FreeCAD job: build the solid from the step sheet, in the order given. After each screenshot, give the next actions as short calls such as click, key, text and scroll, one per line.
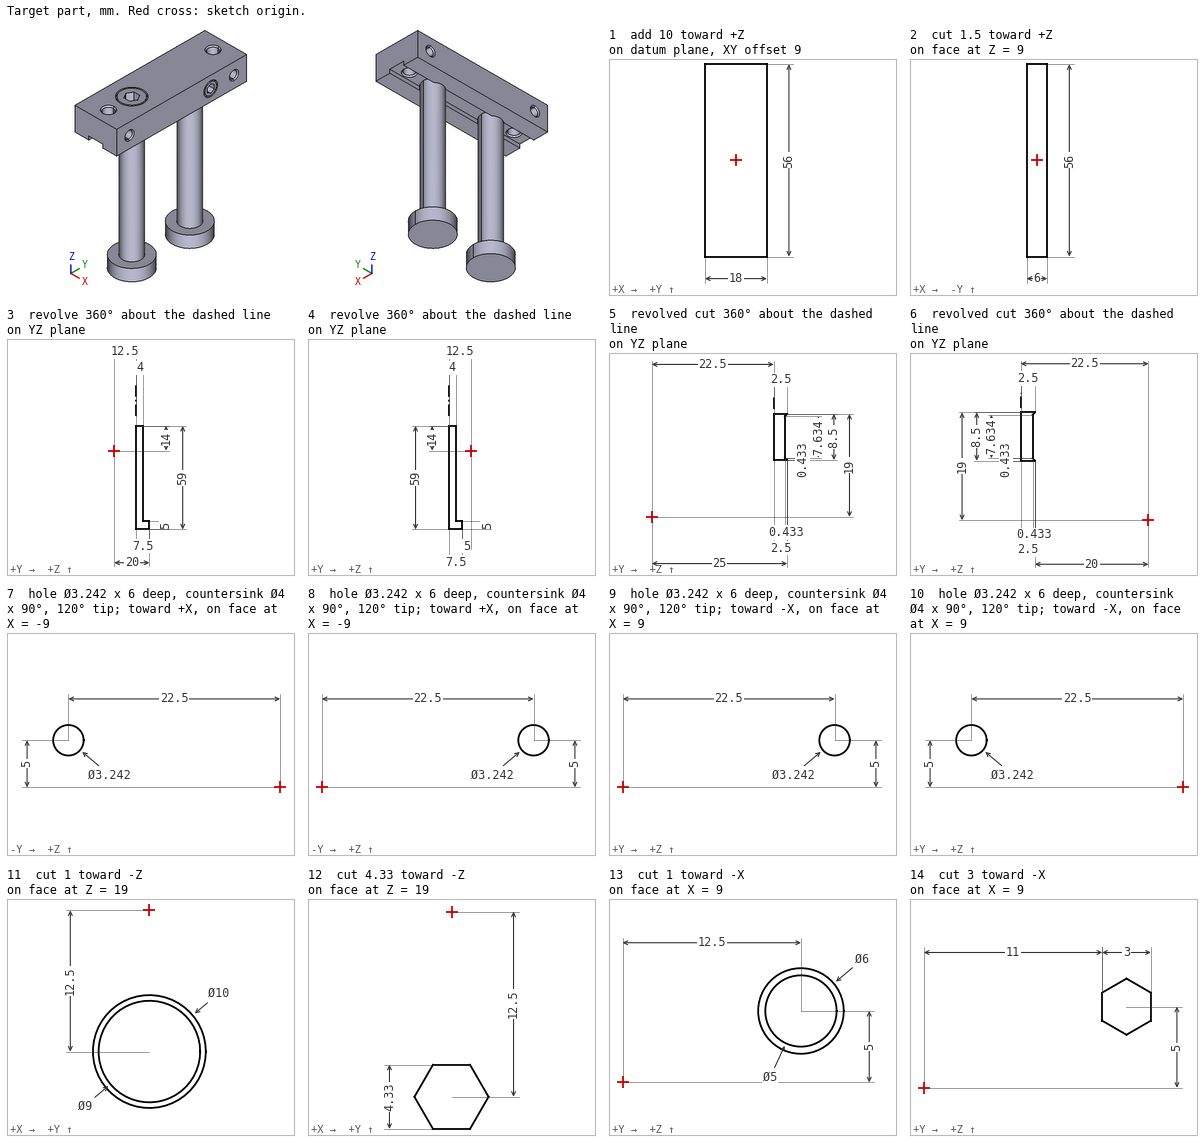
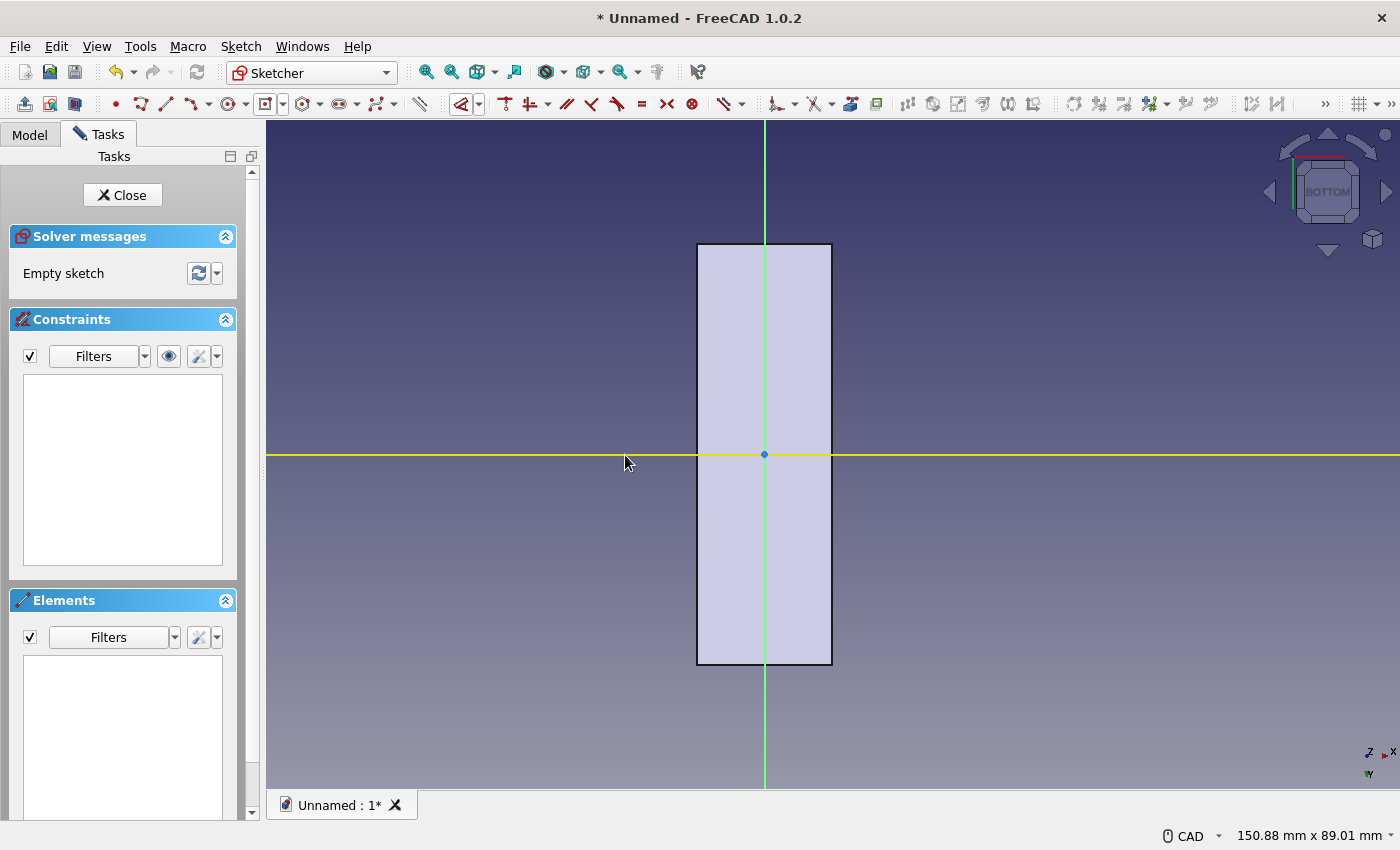
click(264, 104)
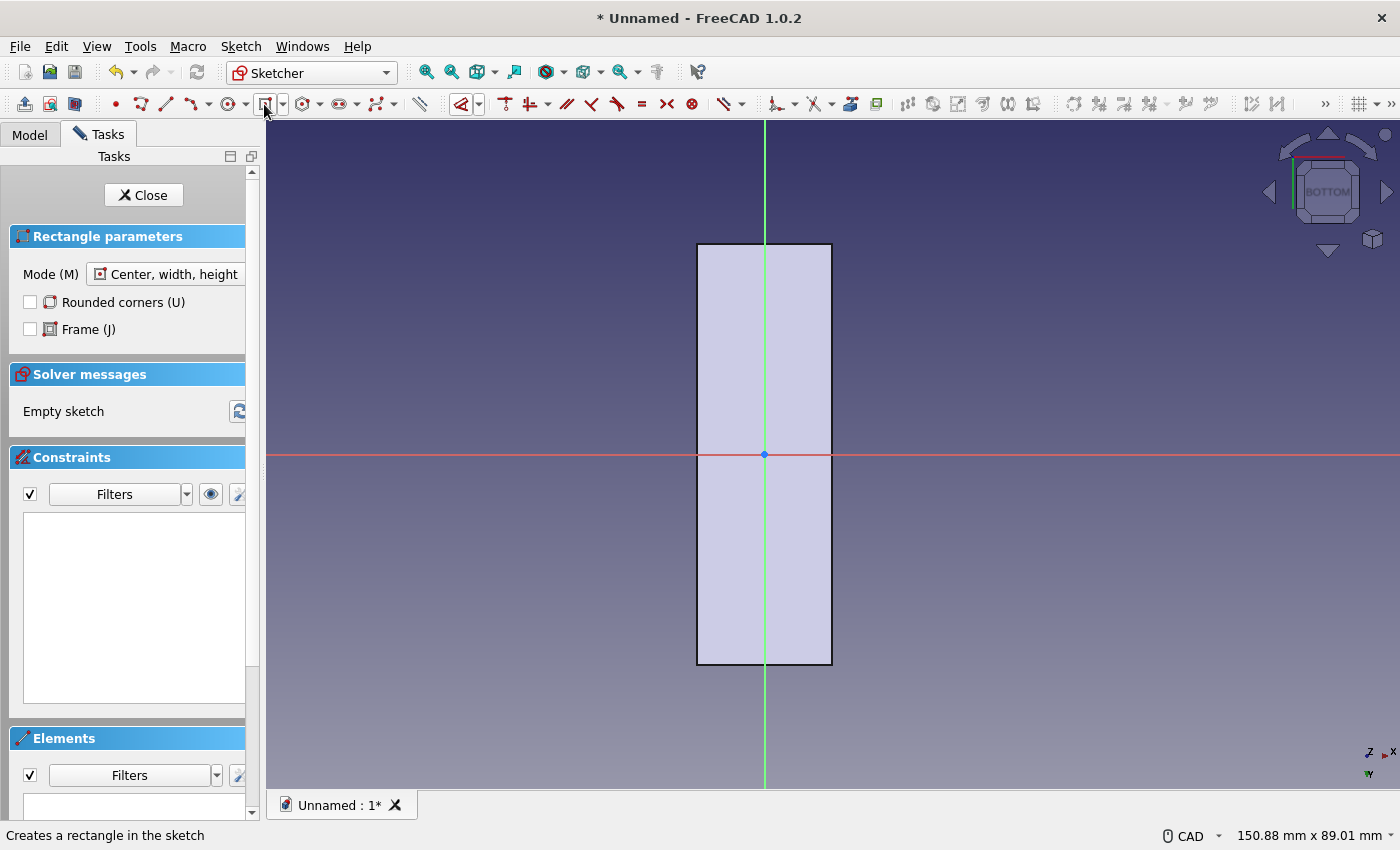
click(765, 455)
move(787, 244)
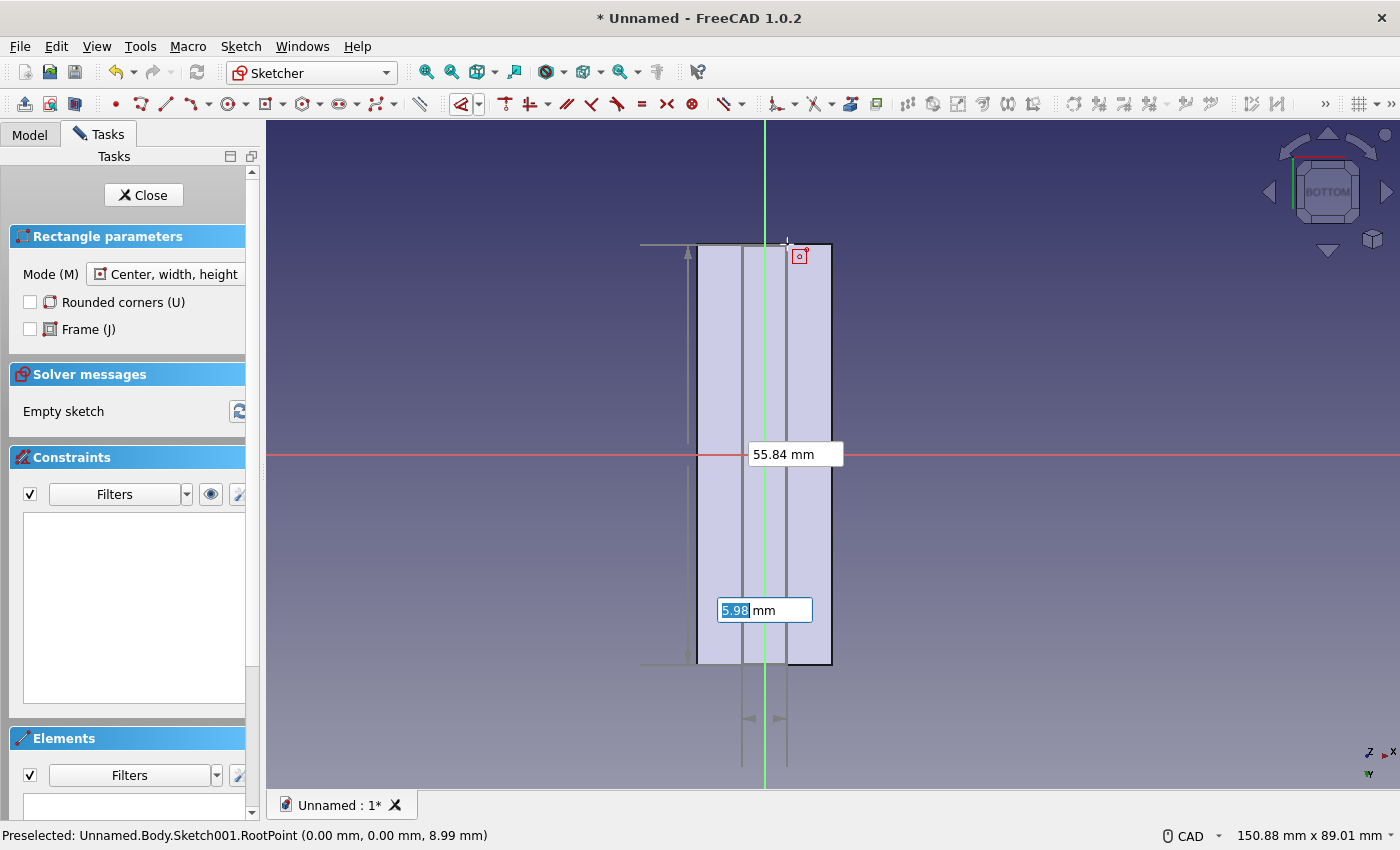
text(6)
key(Tab)
text(56)
key(Return)
key(Escape)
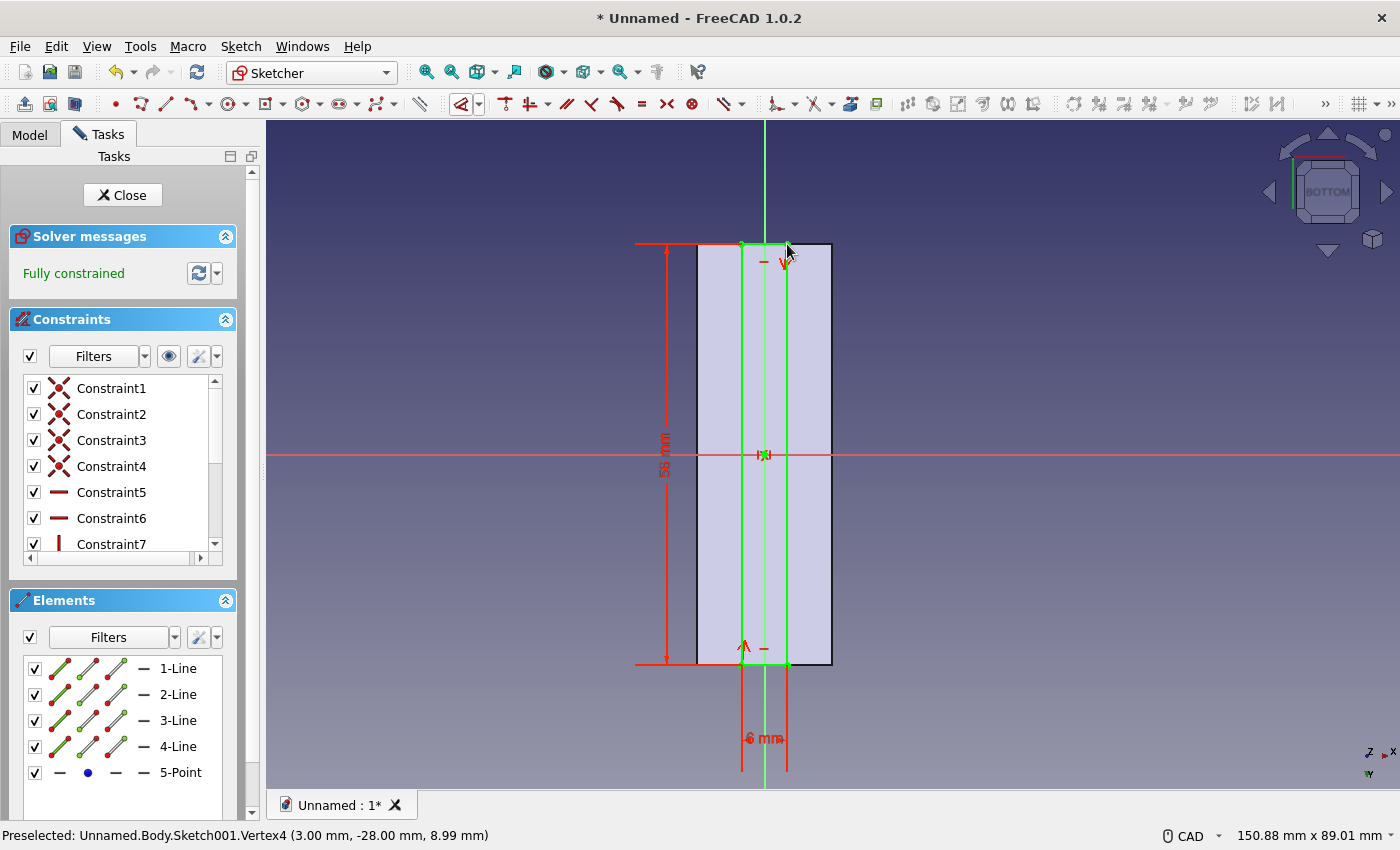
click(123, 195)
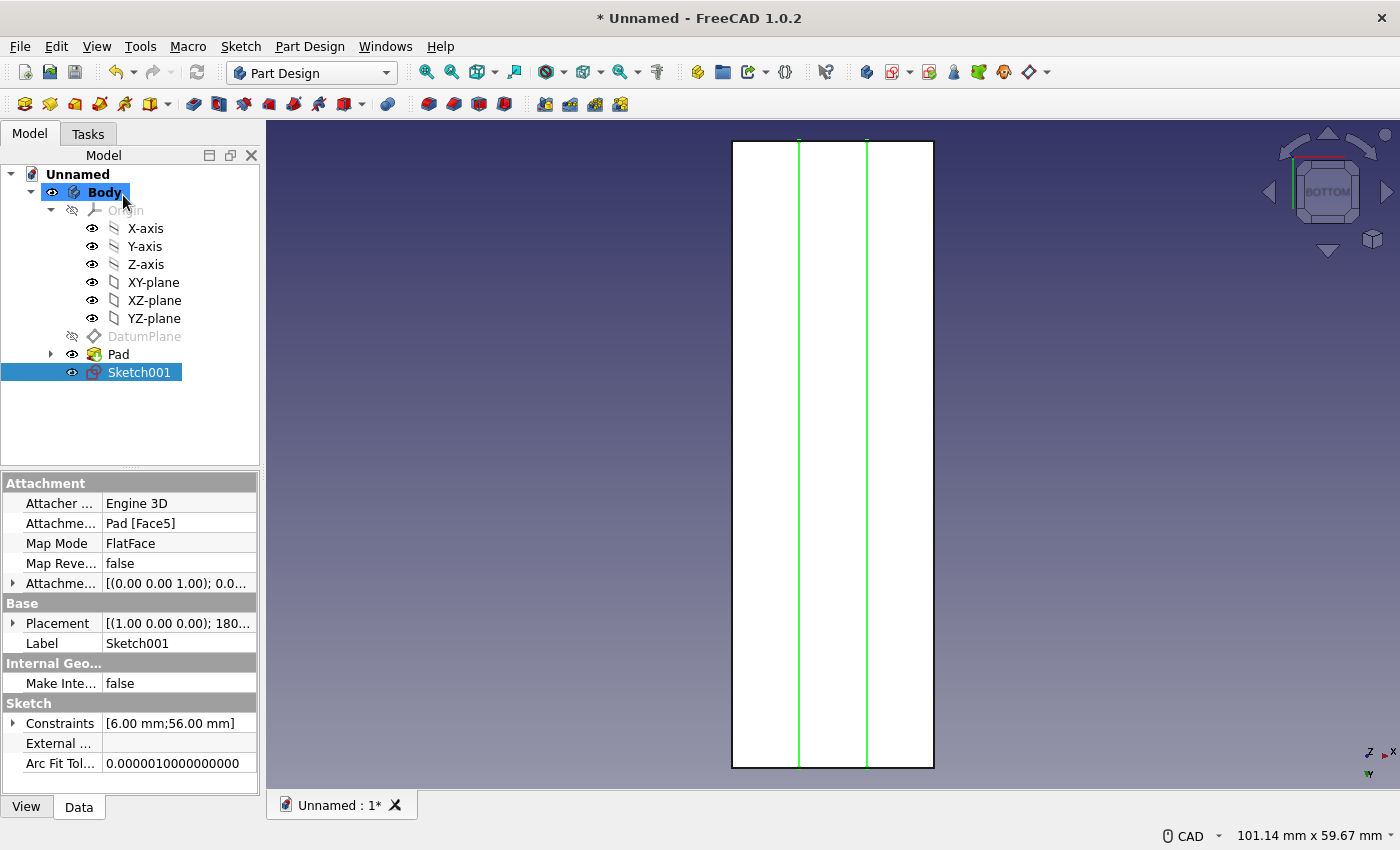
click(194, 104)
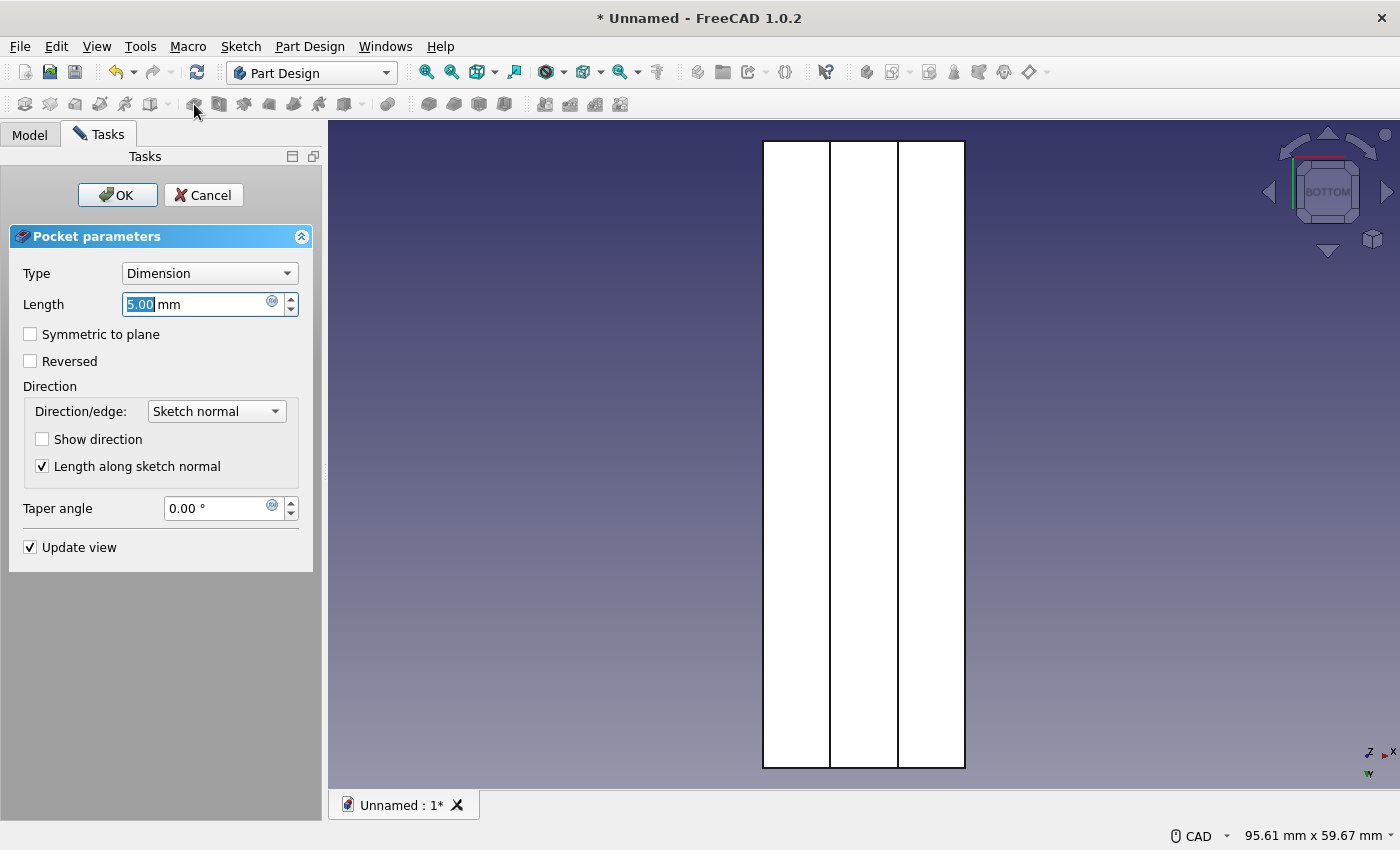
text(1.5)
key(Tab)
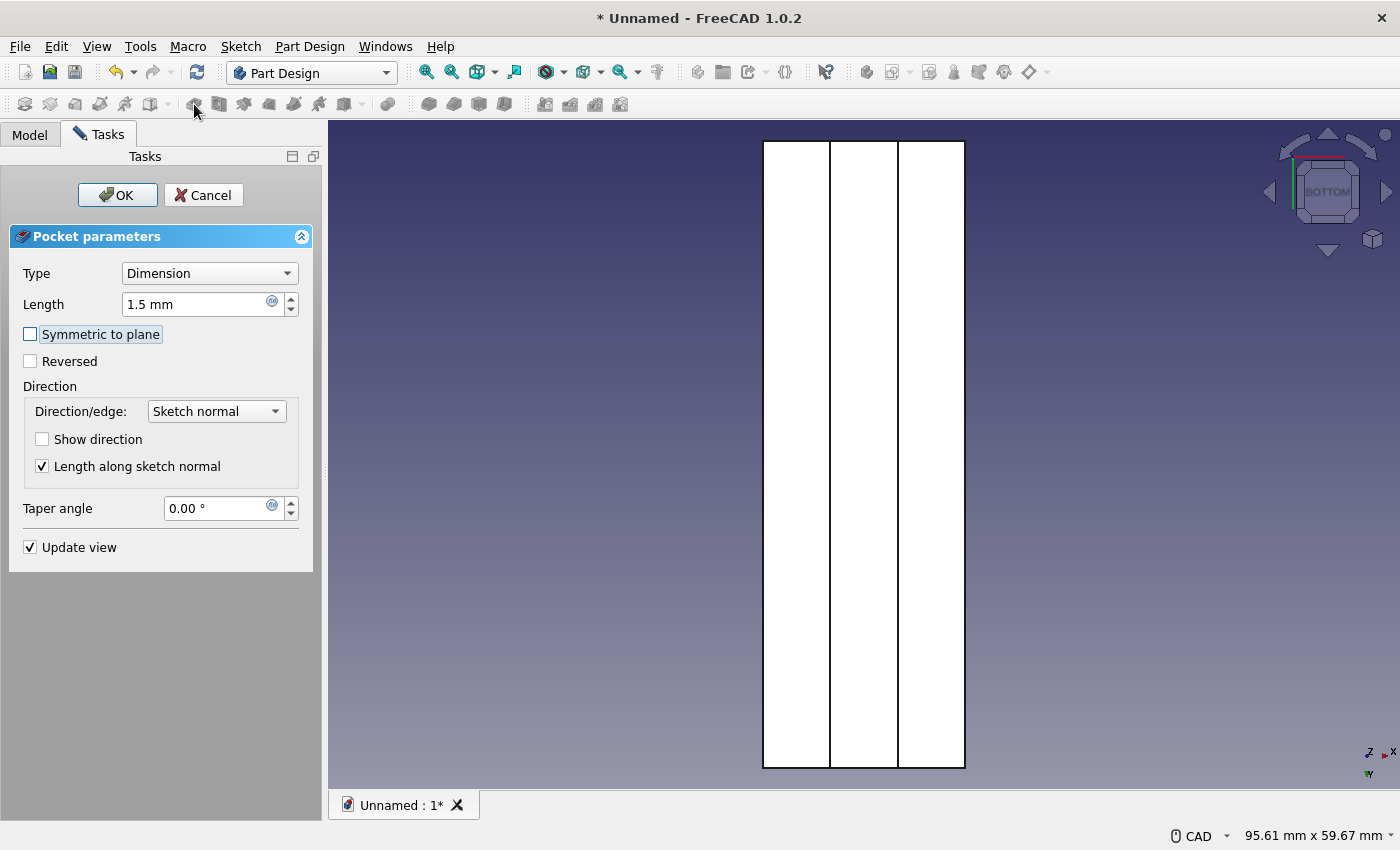
click(118, 195)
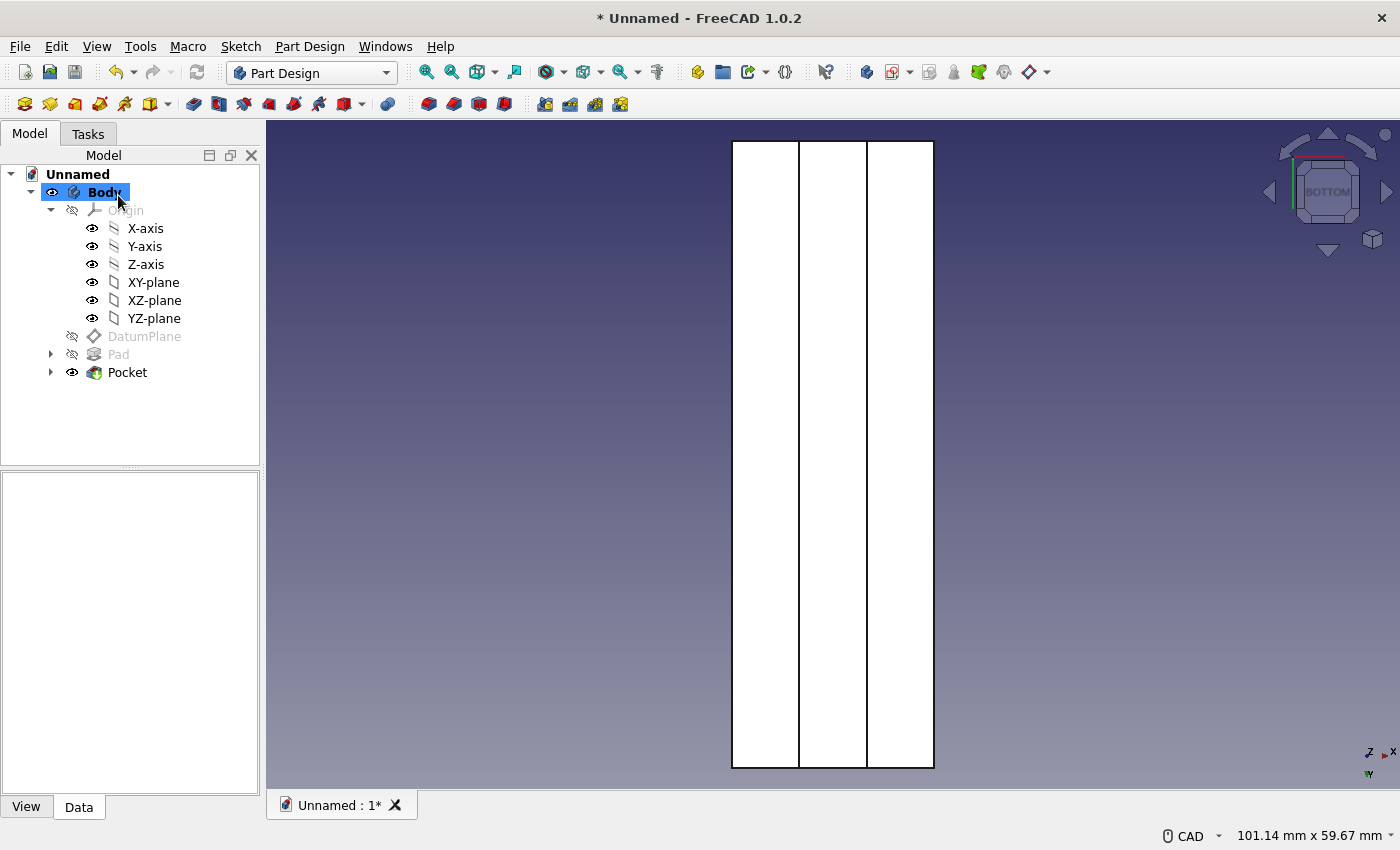
click(892, 72)